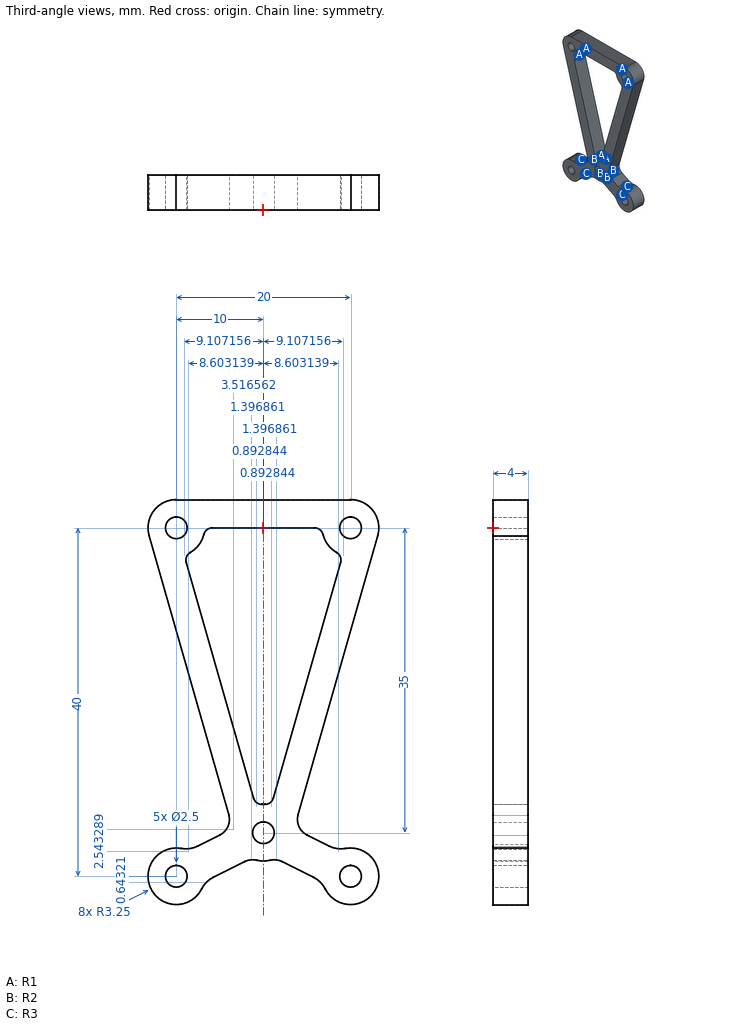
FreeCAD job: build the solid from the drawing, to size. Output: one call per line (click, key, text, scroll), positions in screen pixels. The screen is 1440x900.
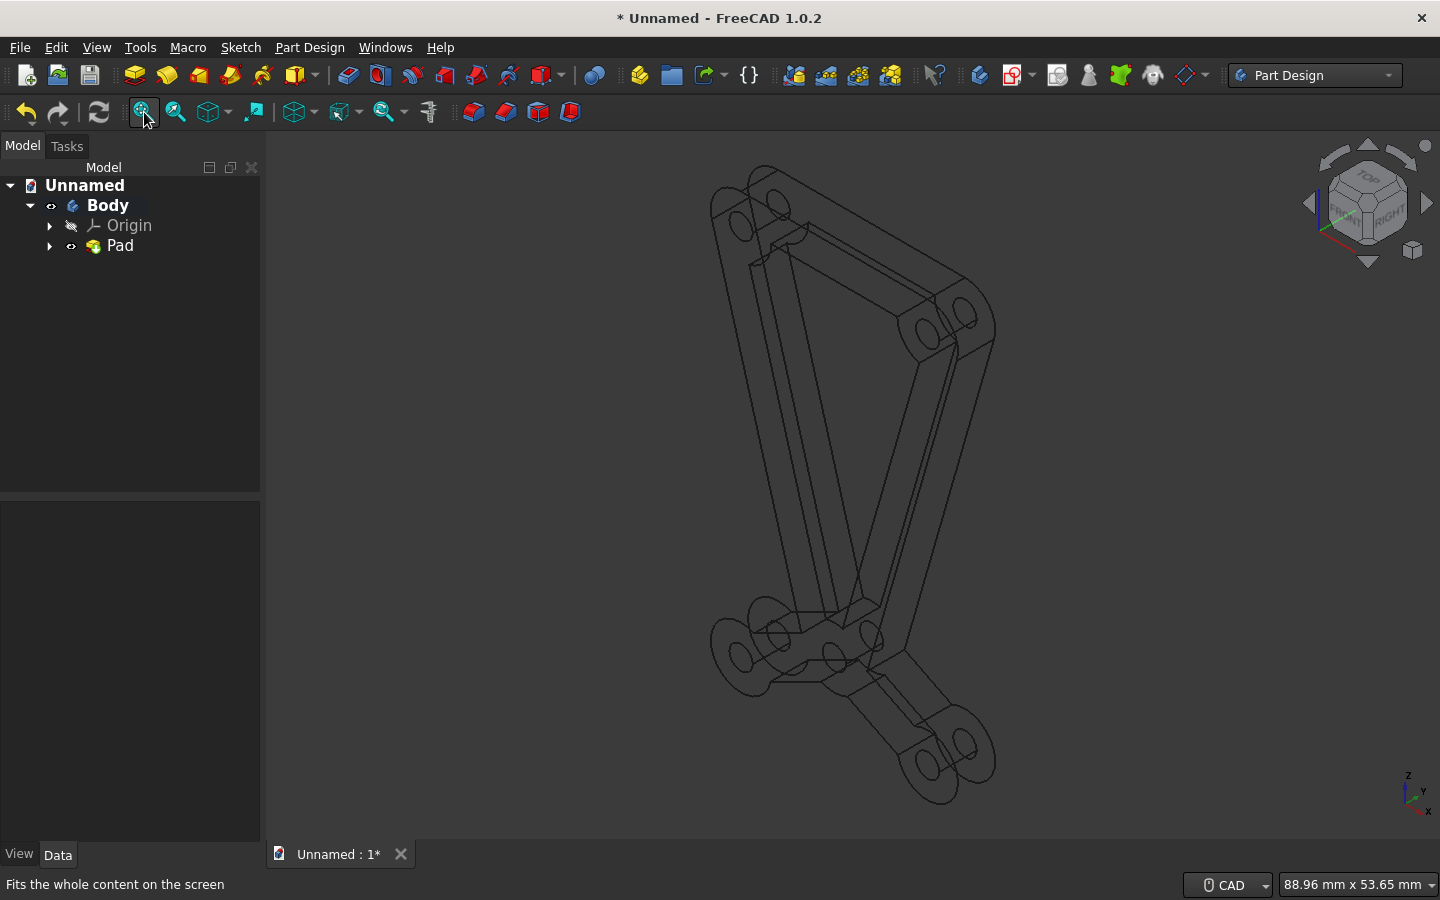
click(931, 356)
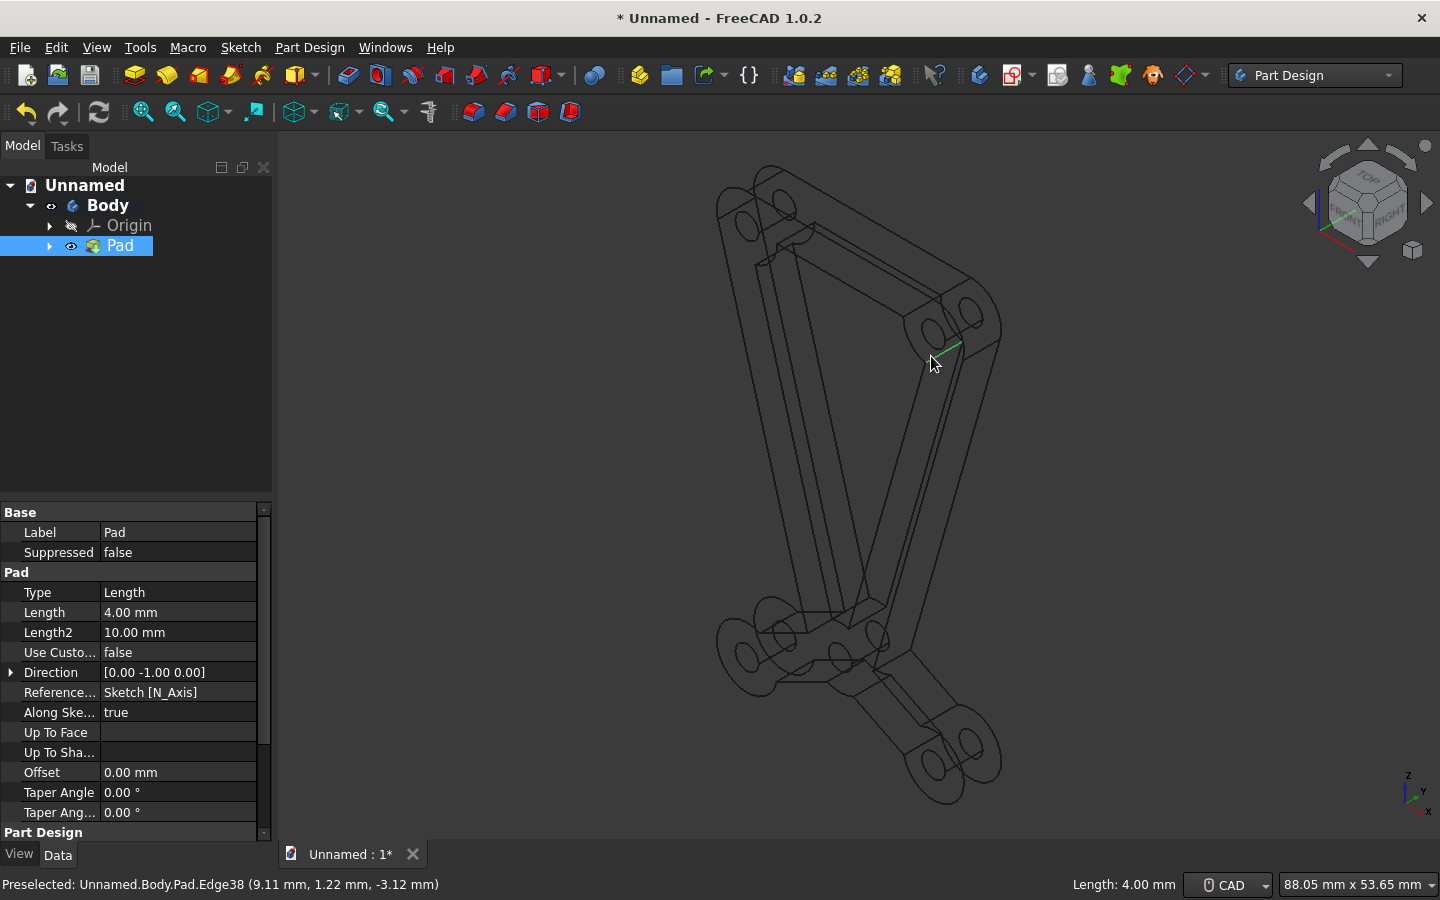
click(867, 617, ctrl)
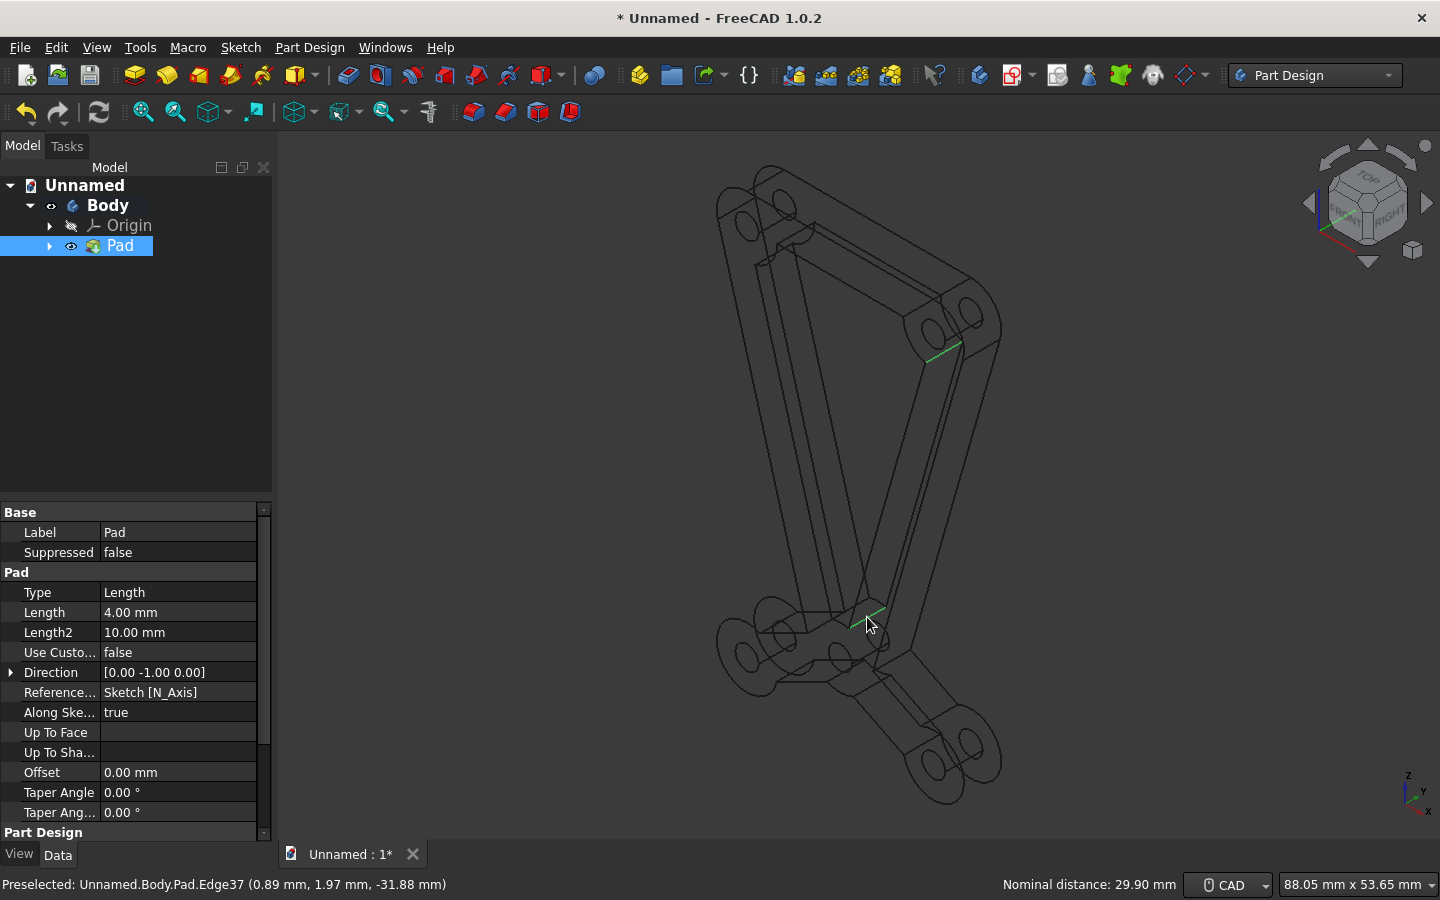
click(847, 609, ctrl)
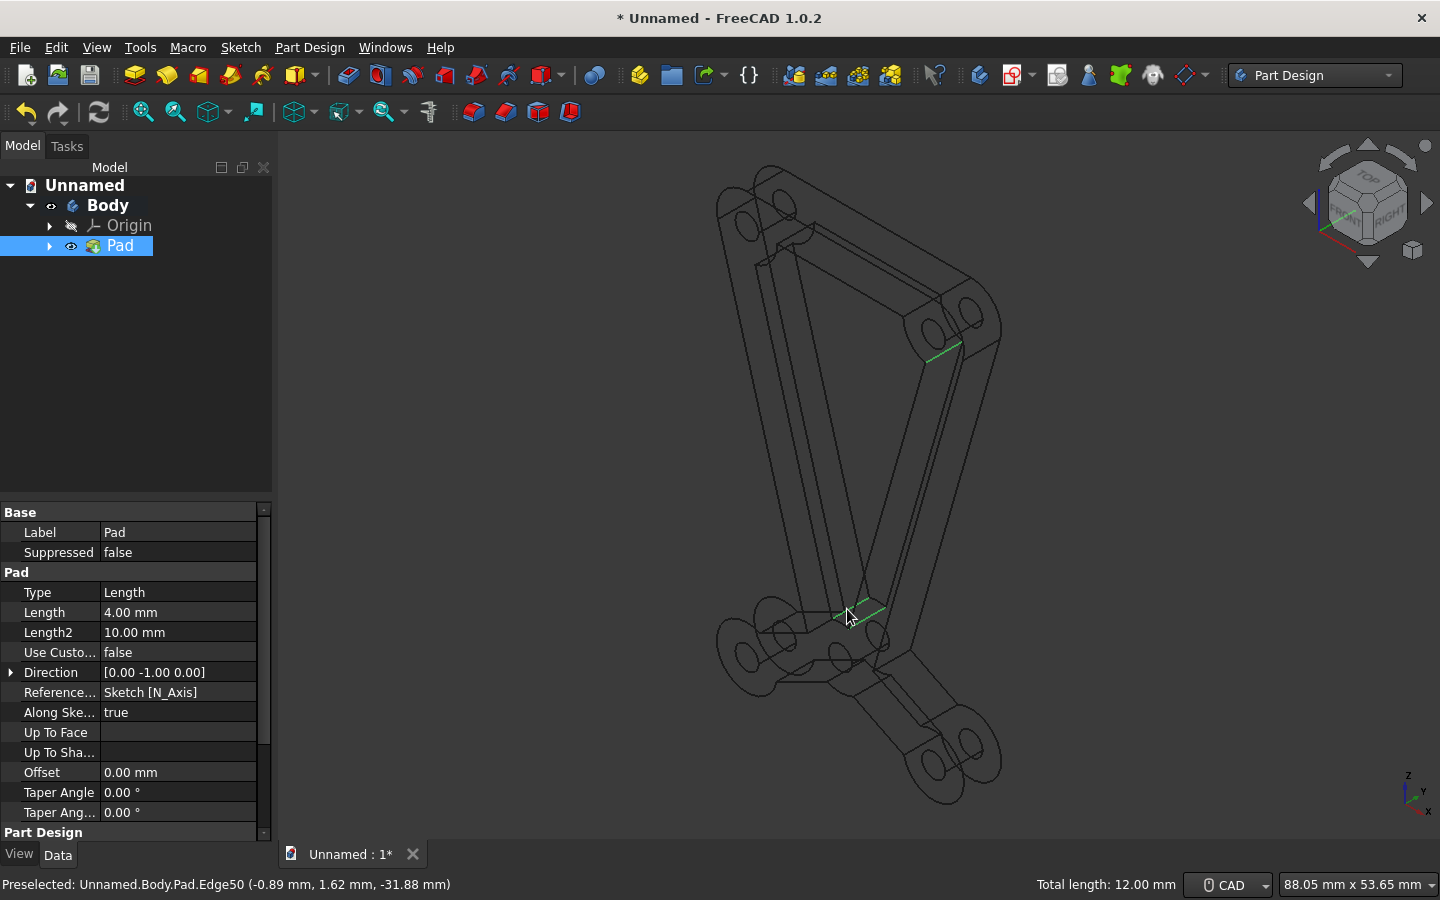
click(796, 232, ctrl)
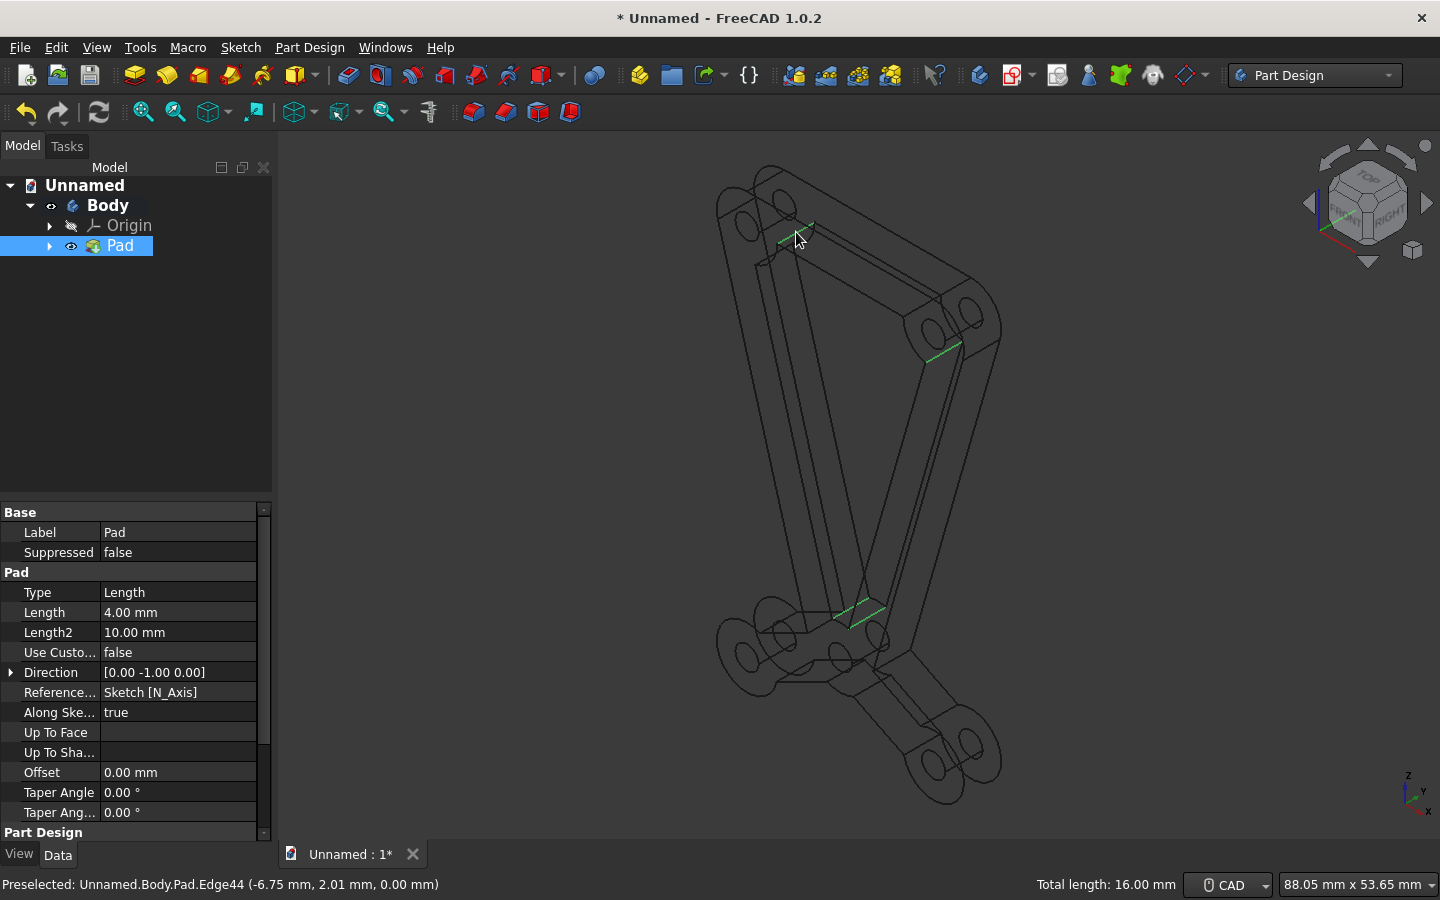
click(922, 305, ctrl)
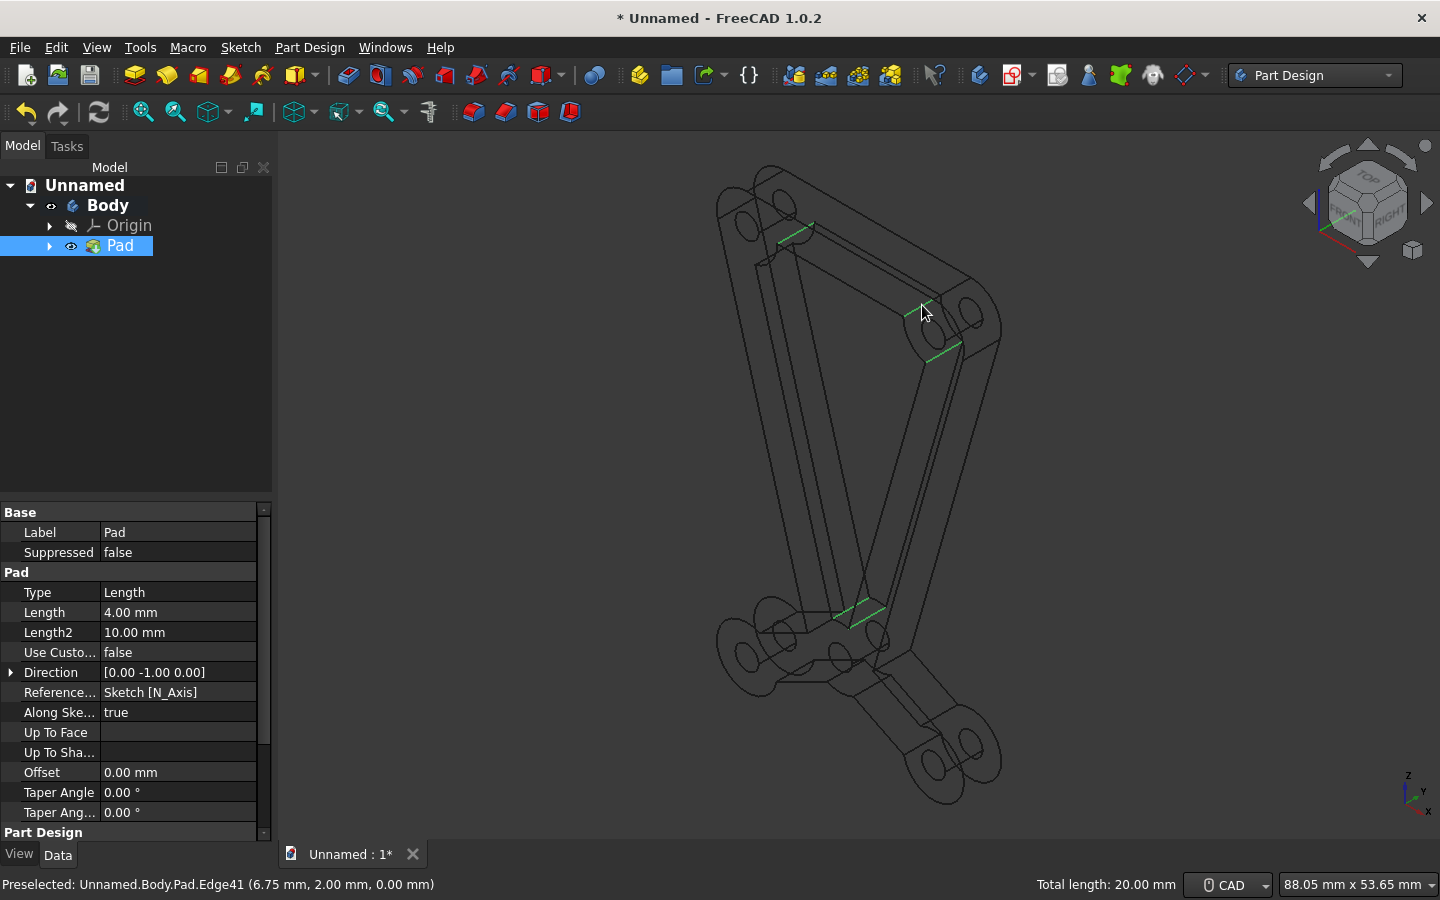
scroll(774, 253, up, 6)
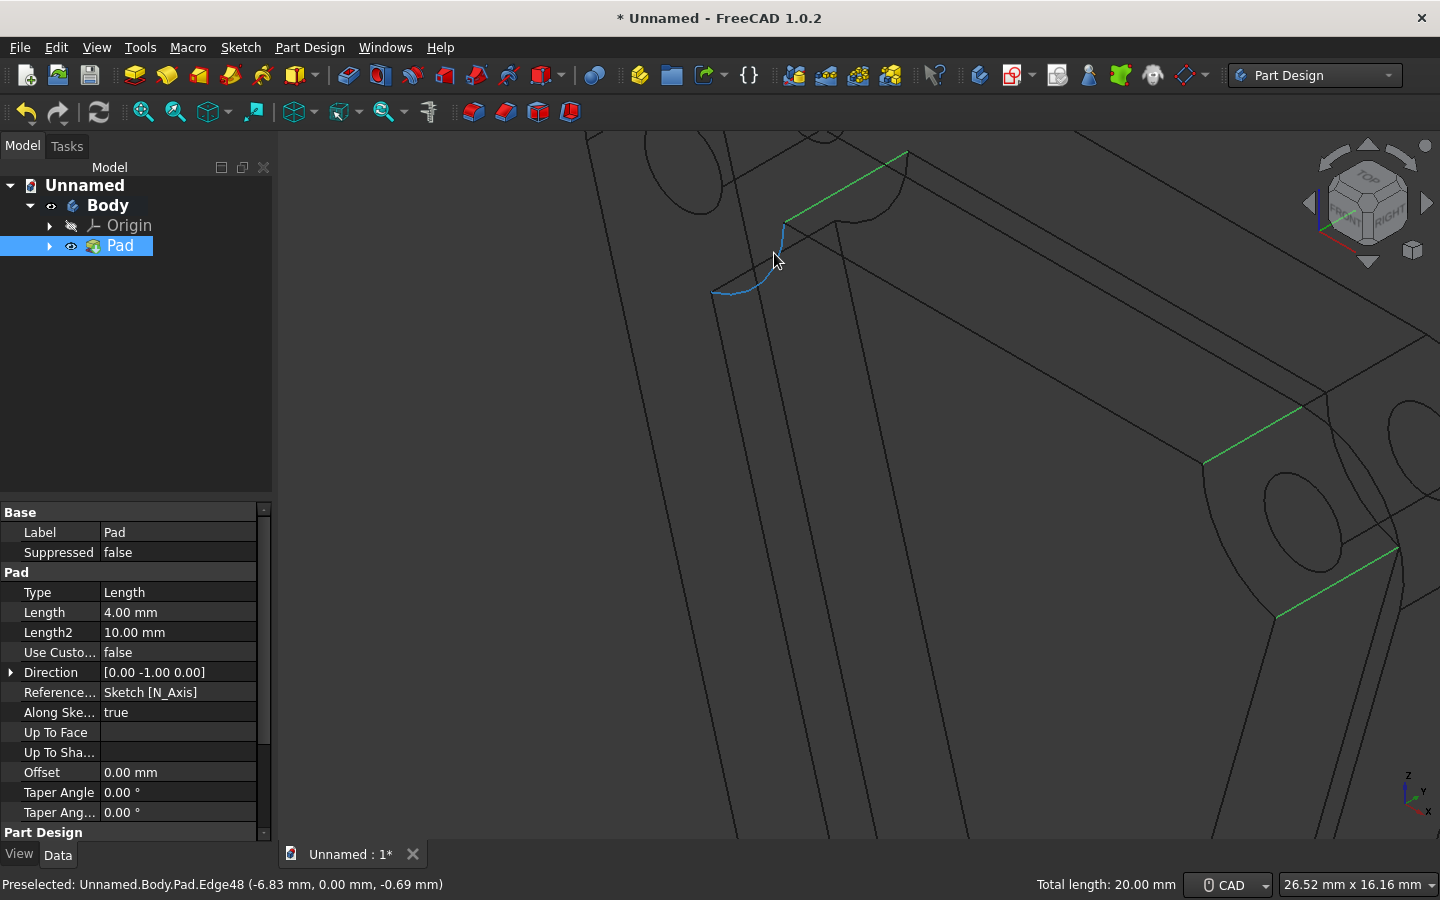
click(761, 263, ctrl)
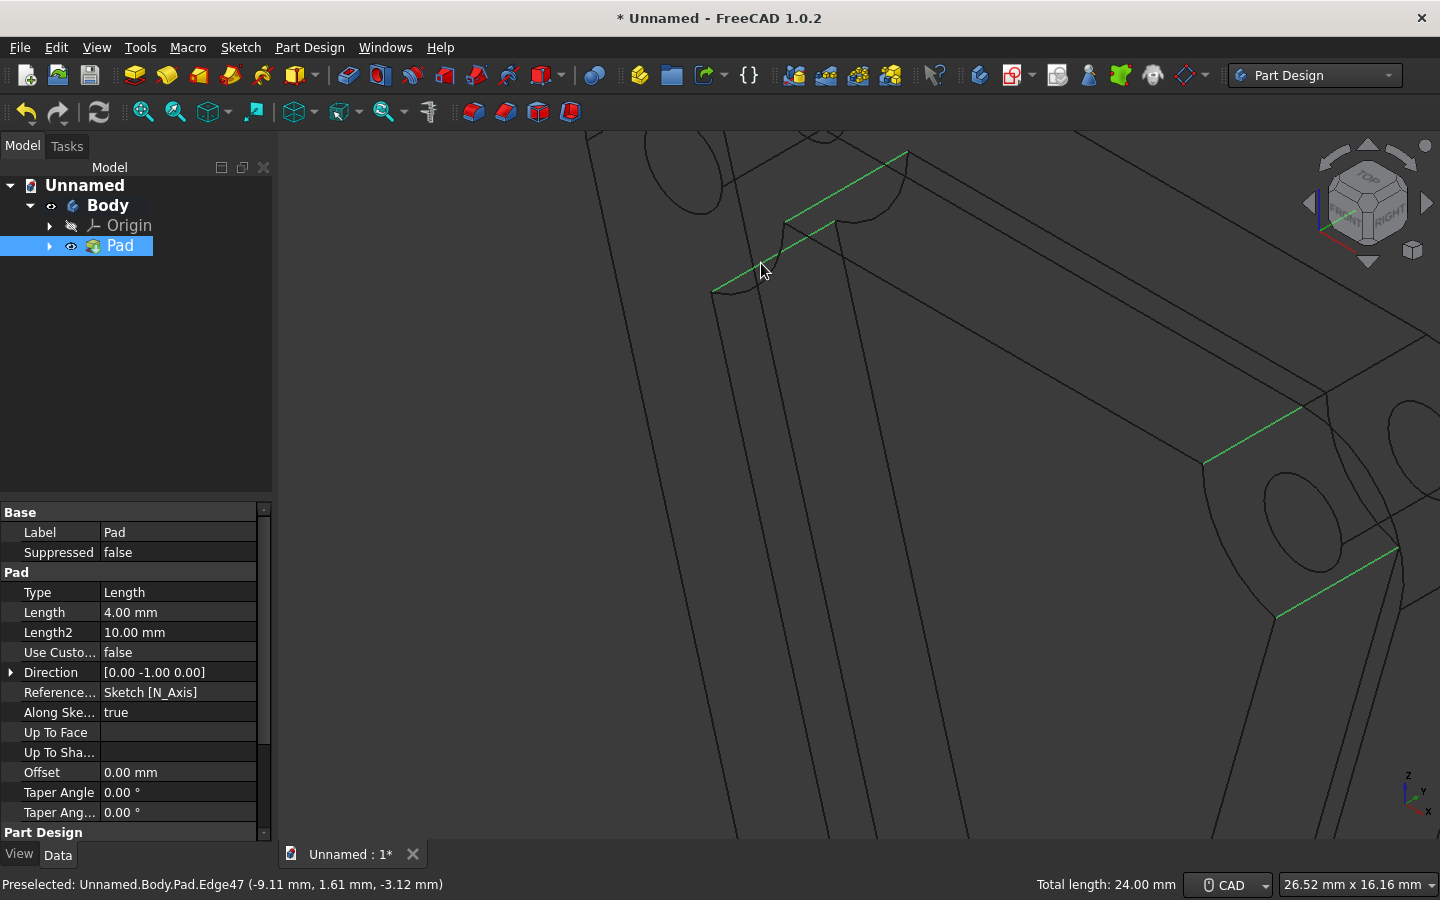
key(v)
key(1)